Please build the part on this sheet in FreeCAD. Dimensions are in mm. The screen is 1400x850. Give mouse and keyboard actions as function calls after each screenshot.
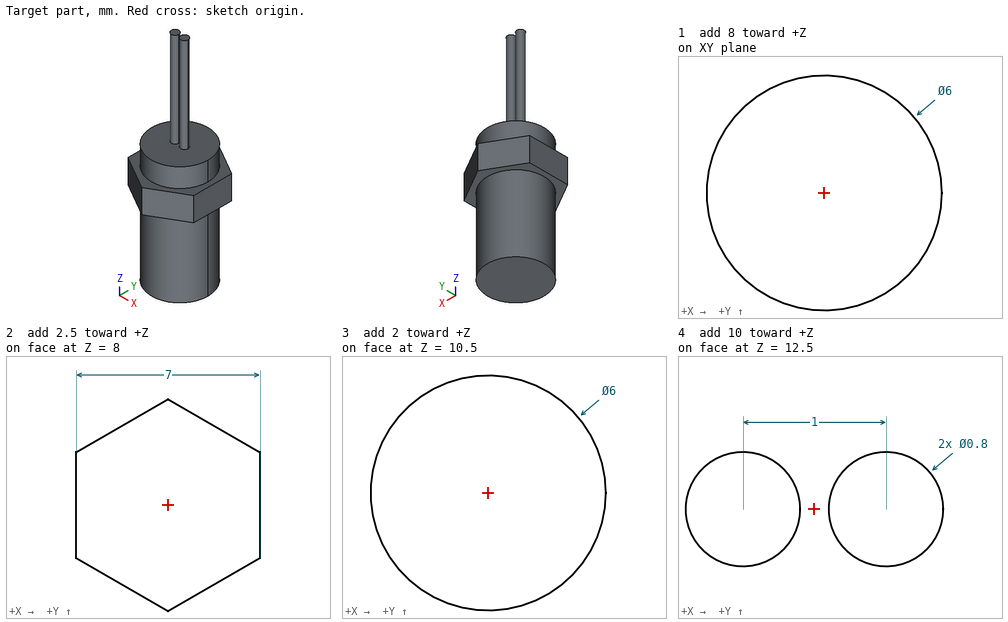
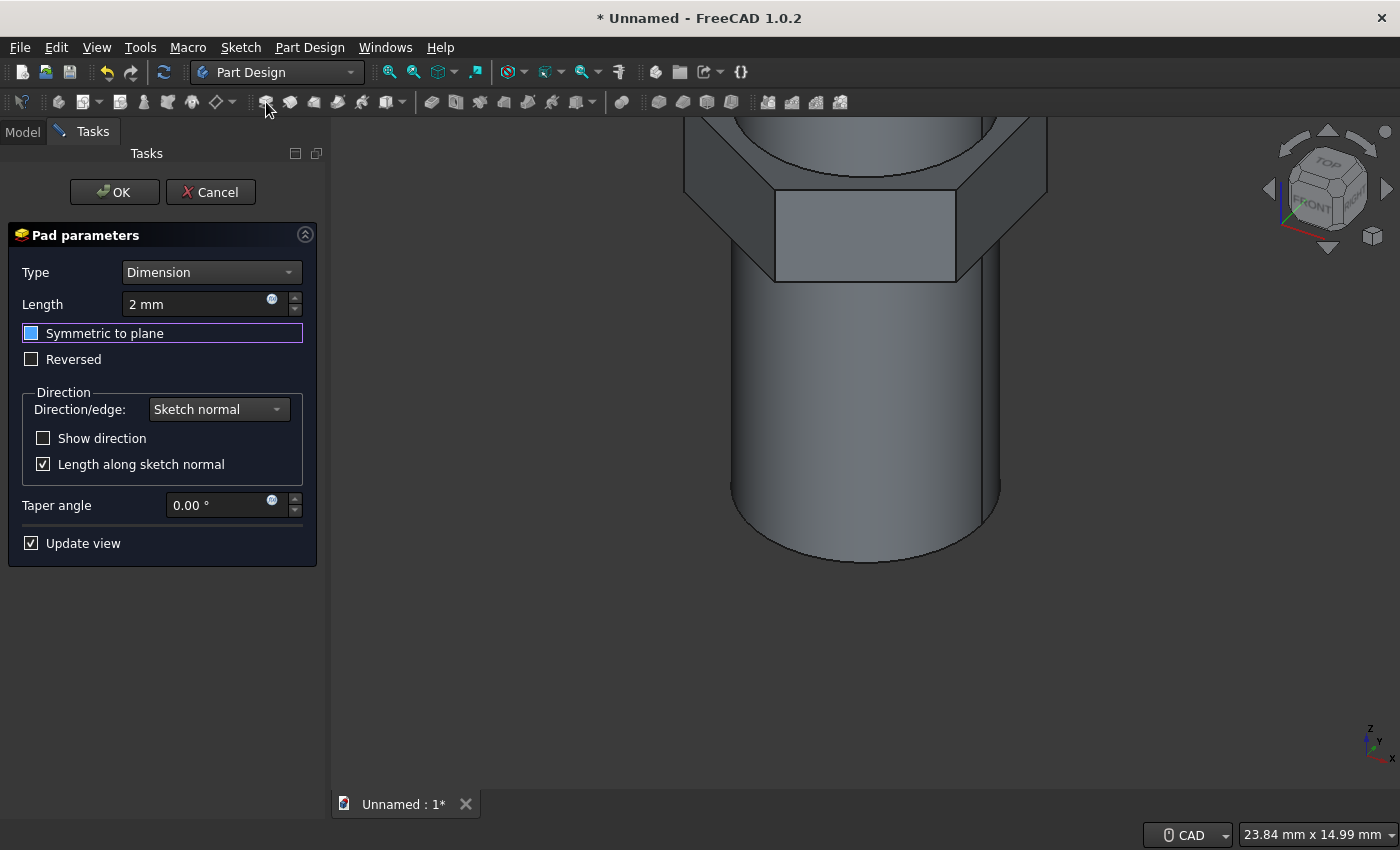
click(115, 192)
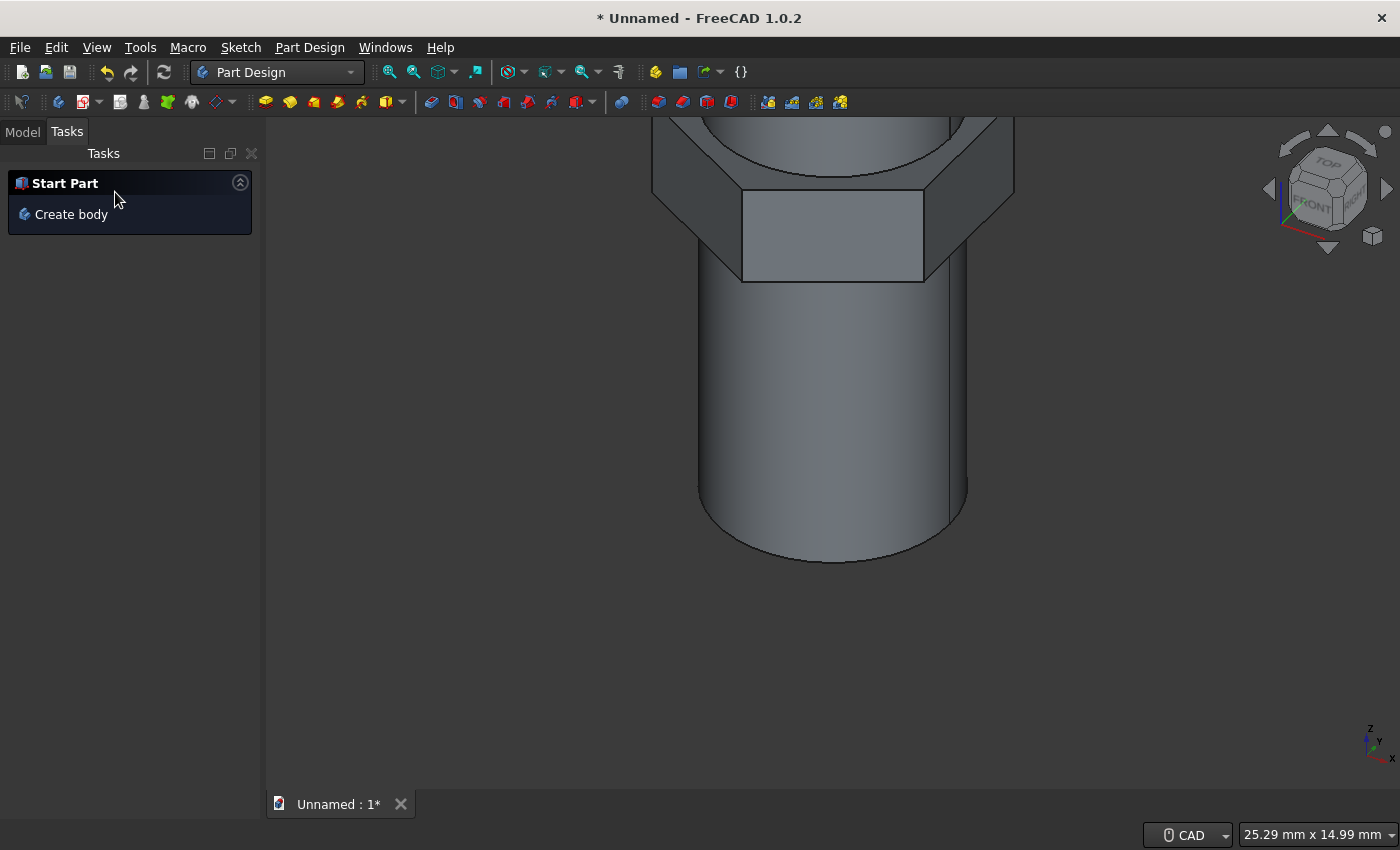
click(390, 72)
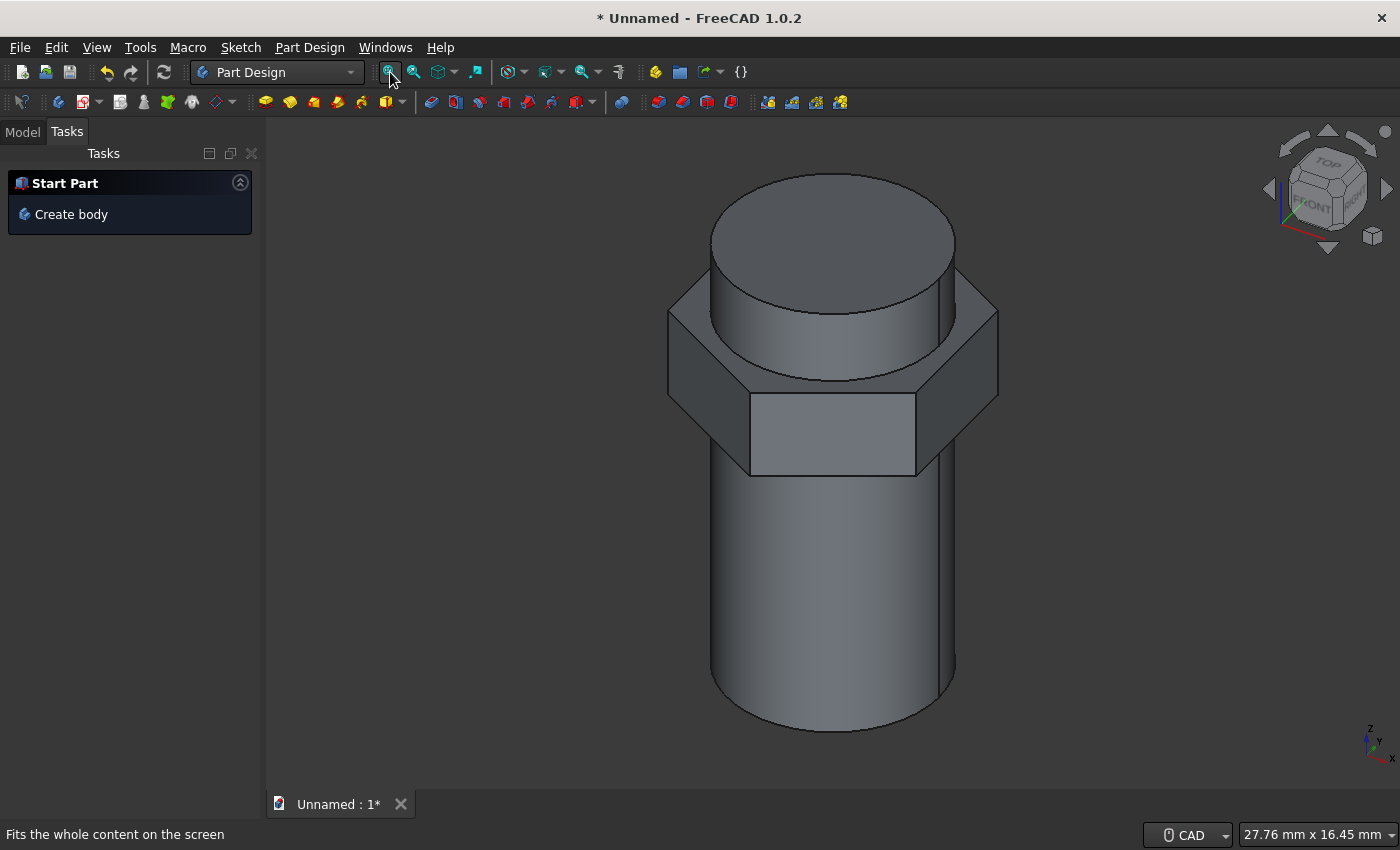
click(833, 243)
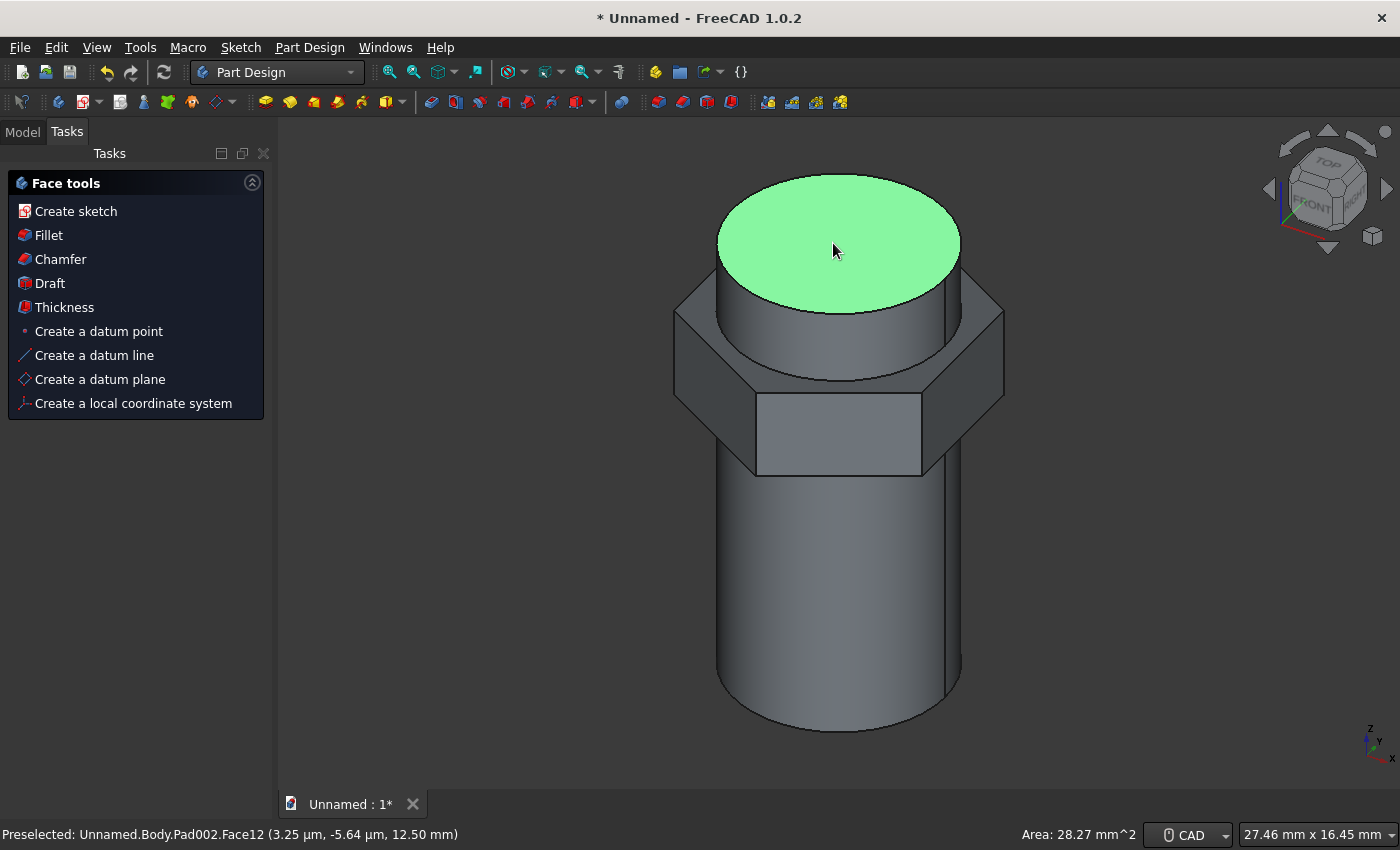
click(84, 102)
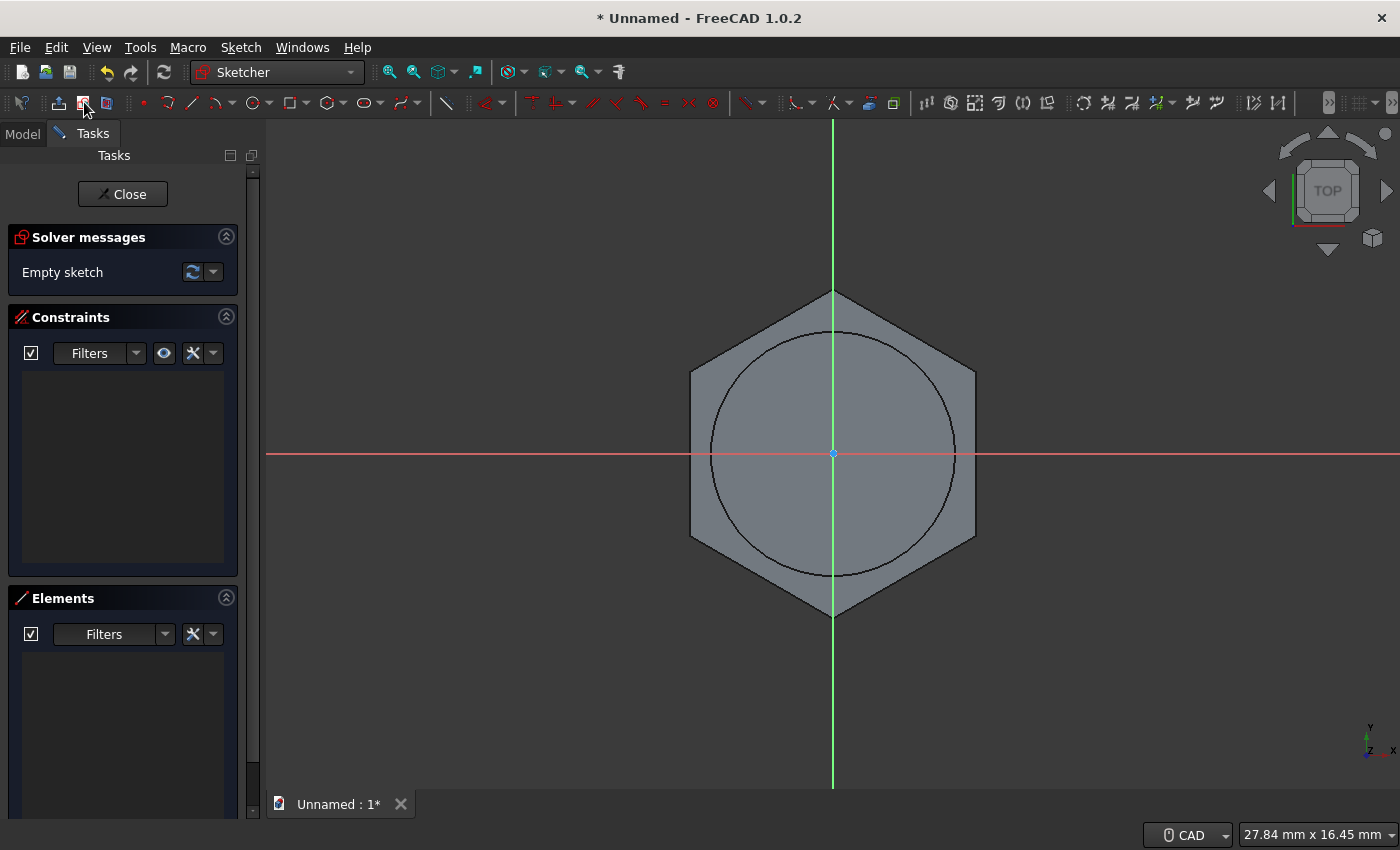
scroll(842, 454, up, 11)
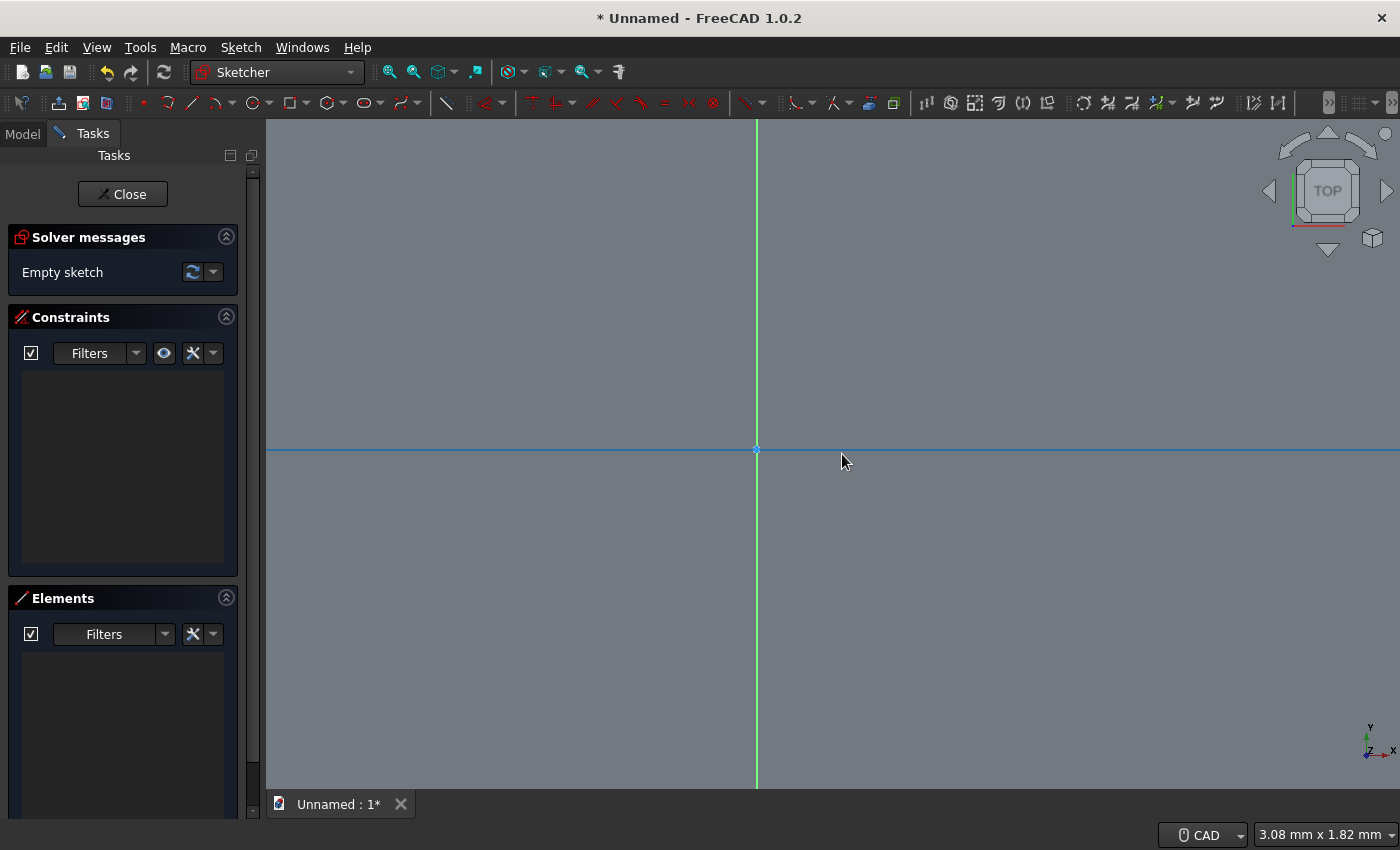
key(g)
key(c)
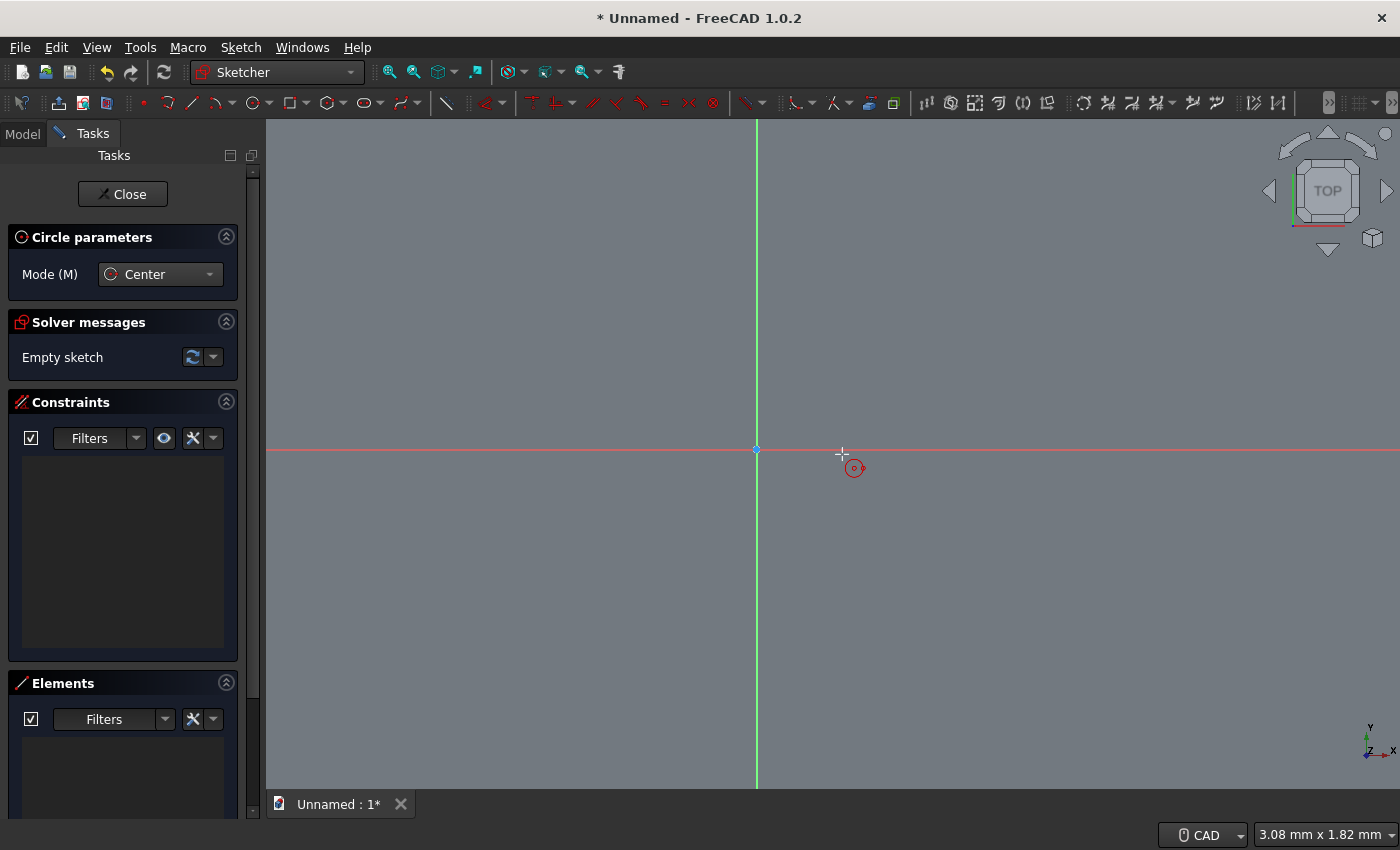
click(940, 450)
move(1044, 346)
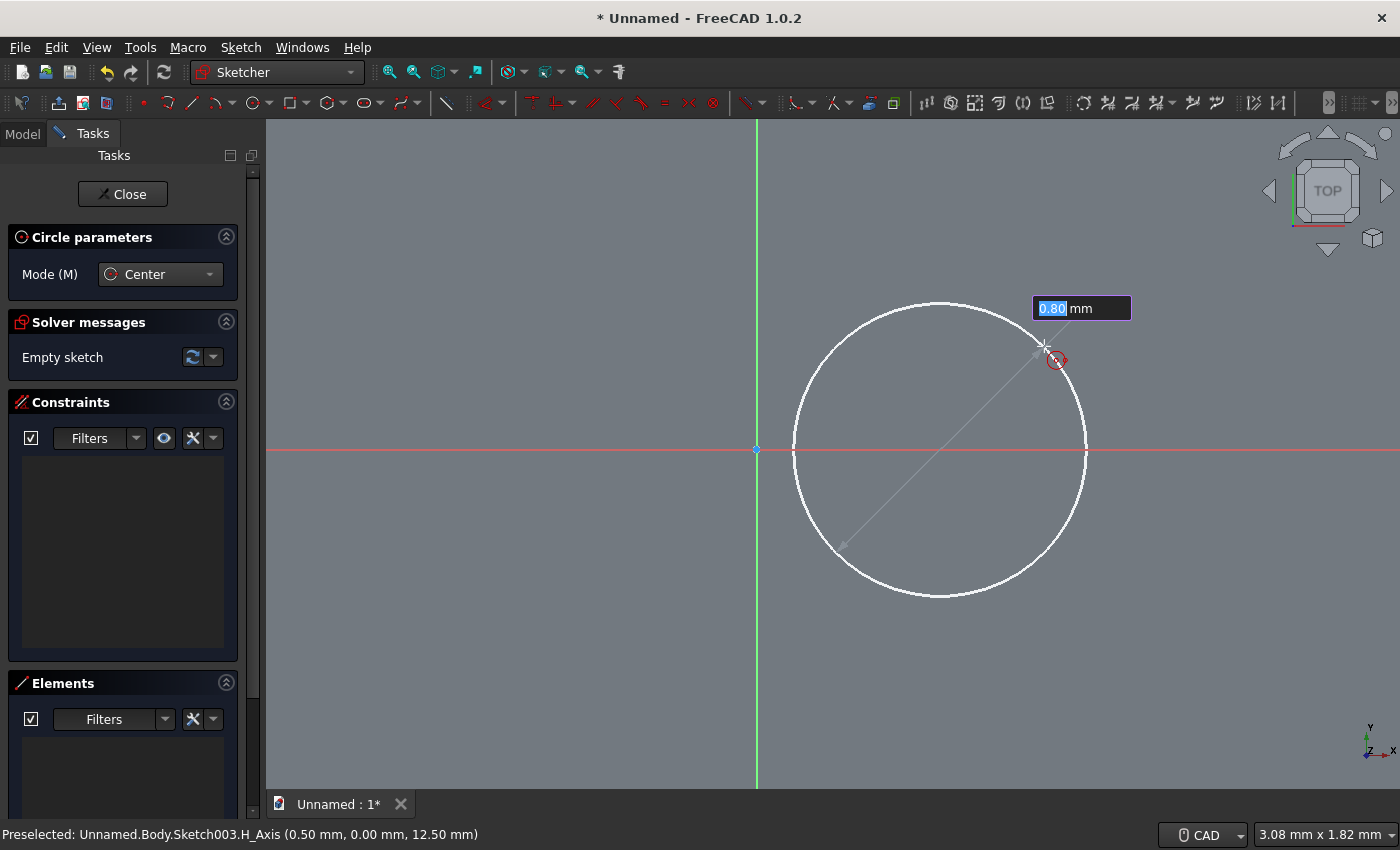
text(0.8)
key(Return)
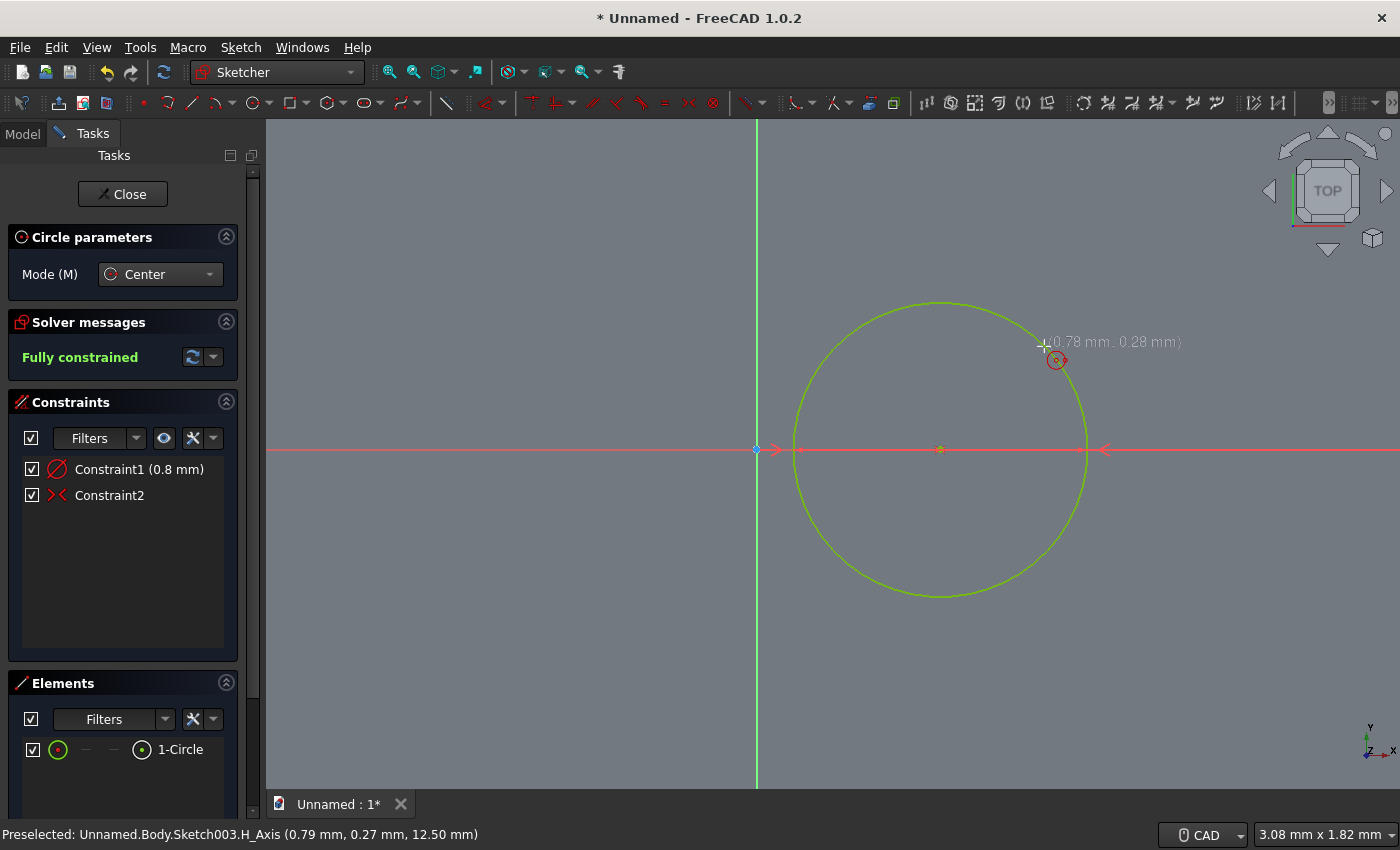
click(573, 450)
move(677, 346)